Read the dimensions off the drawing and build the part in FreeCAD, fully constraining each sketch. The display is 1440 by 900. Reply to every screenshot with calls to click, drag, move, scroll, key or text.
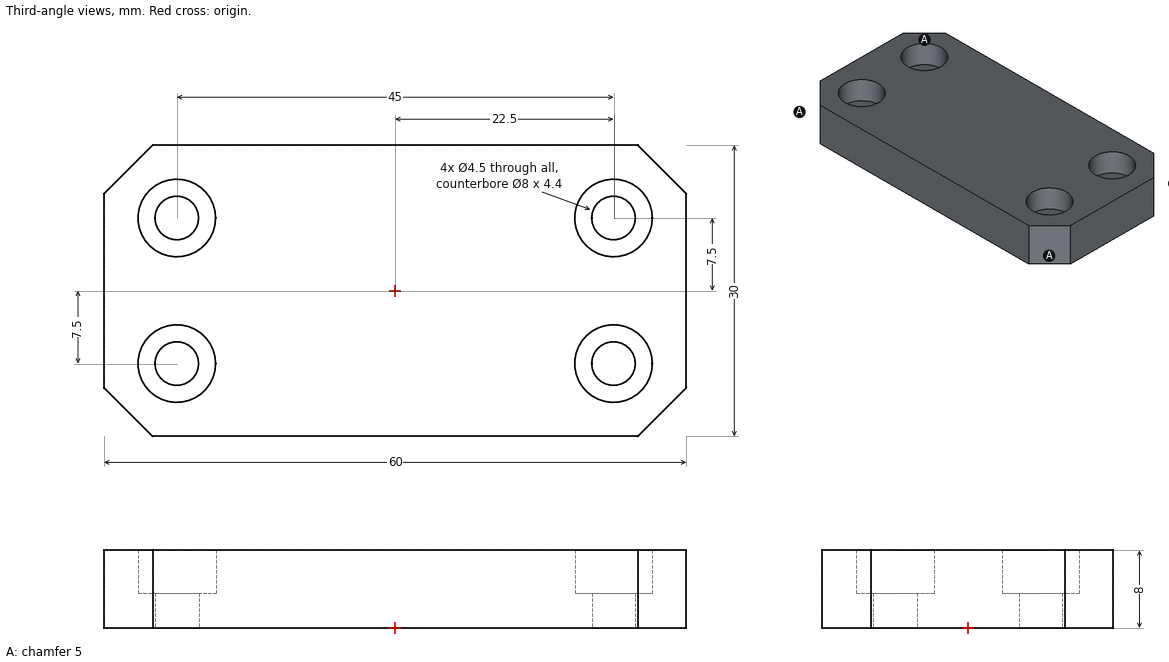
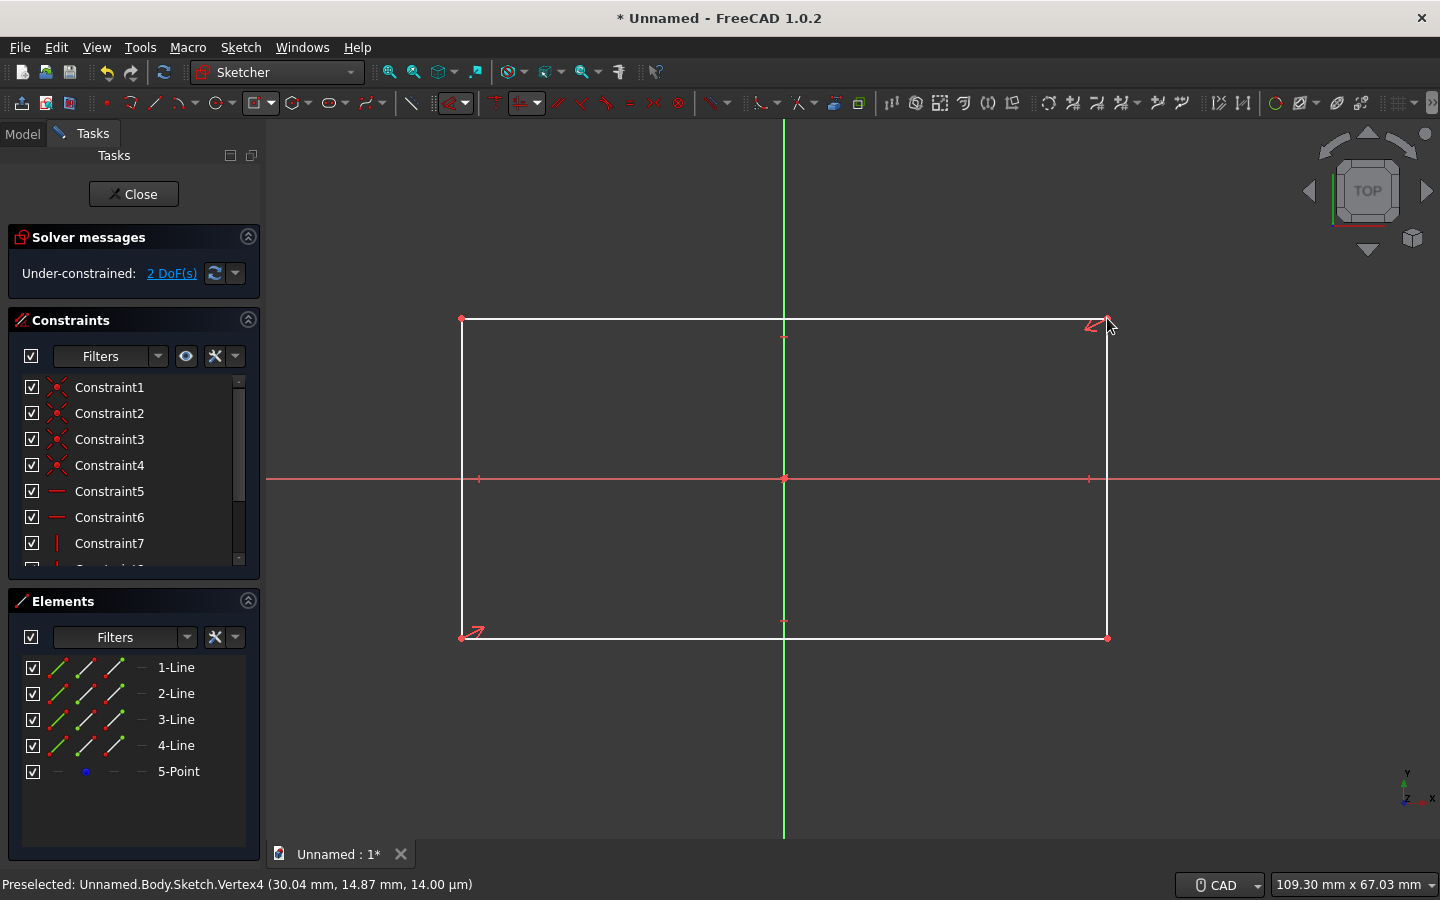
click(450, 104)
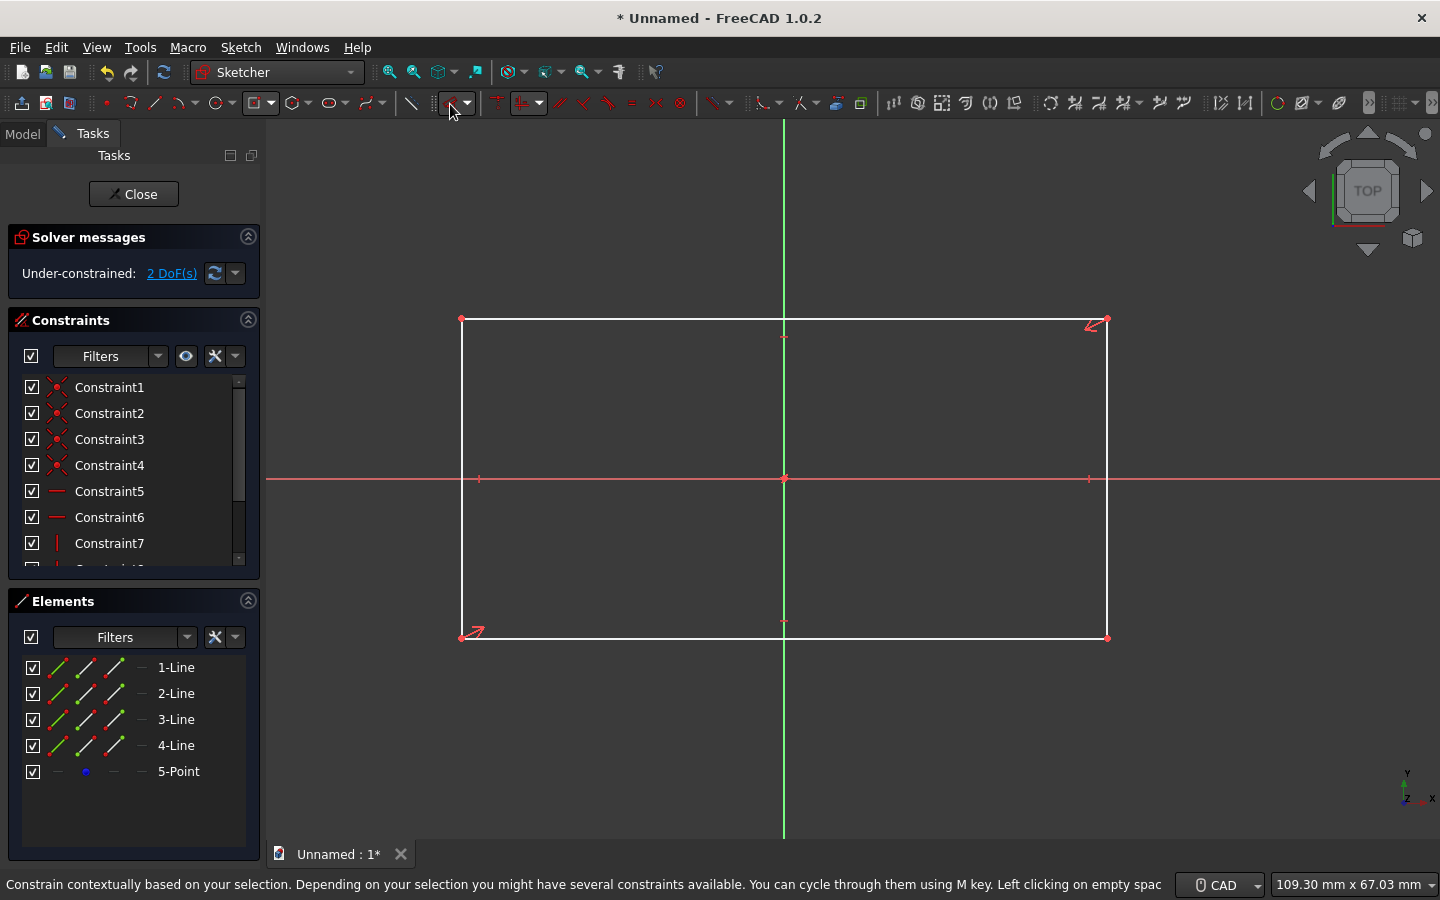
click(655, 639)
click(636, 673)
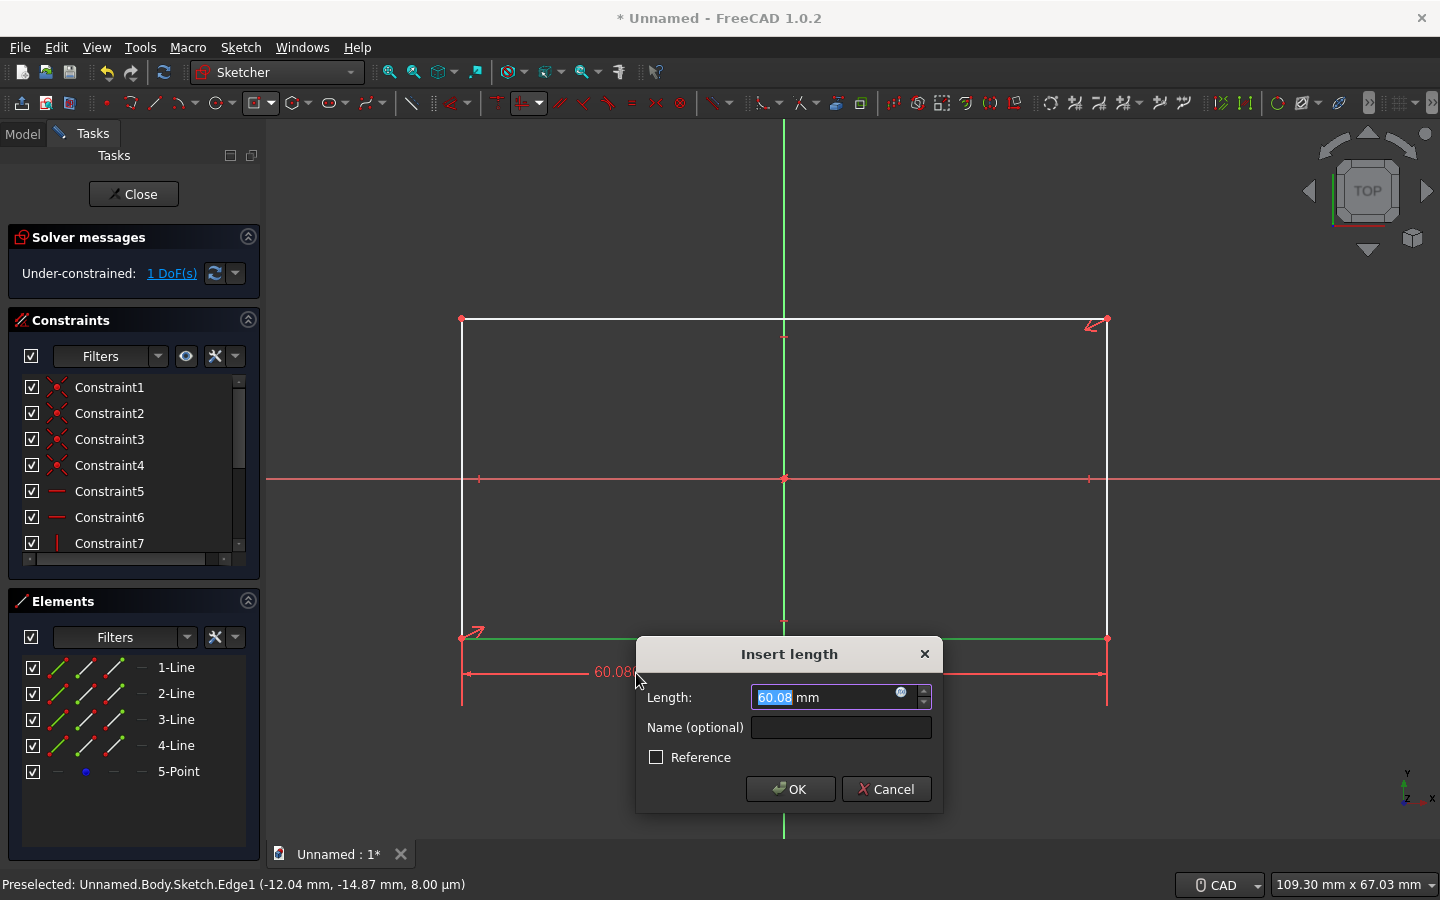
text(60)
key(Return)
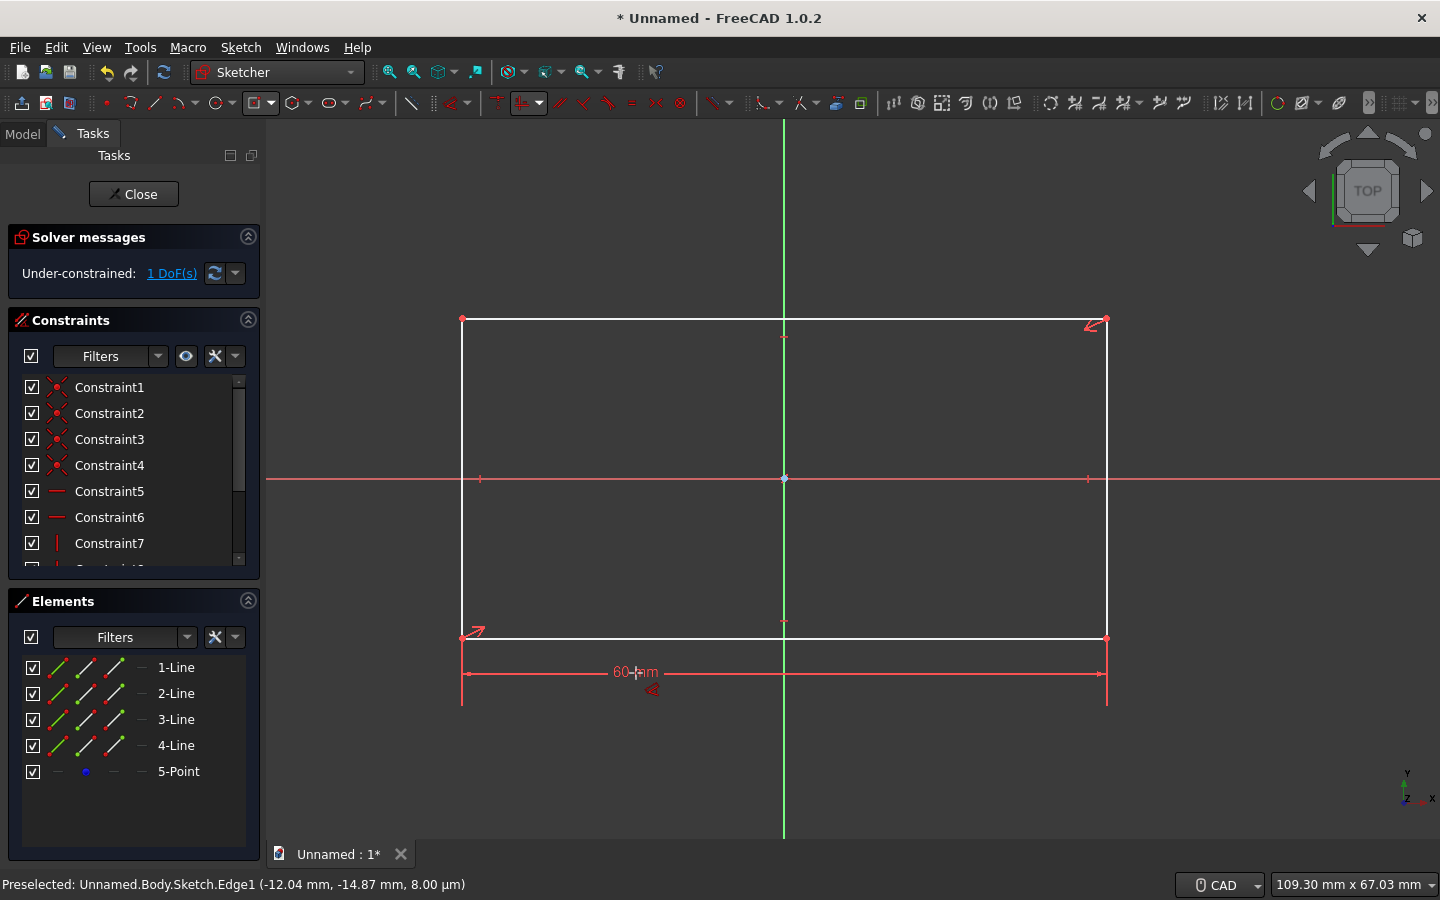
click(1107, 543)
click(1141, 405)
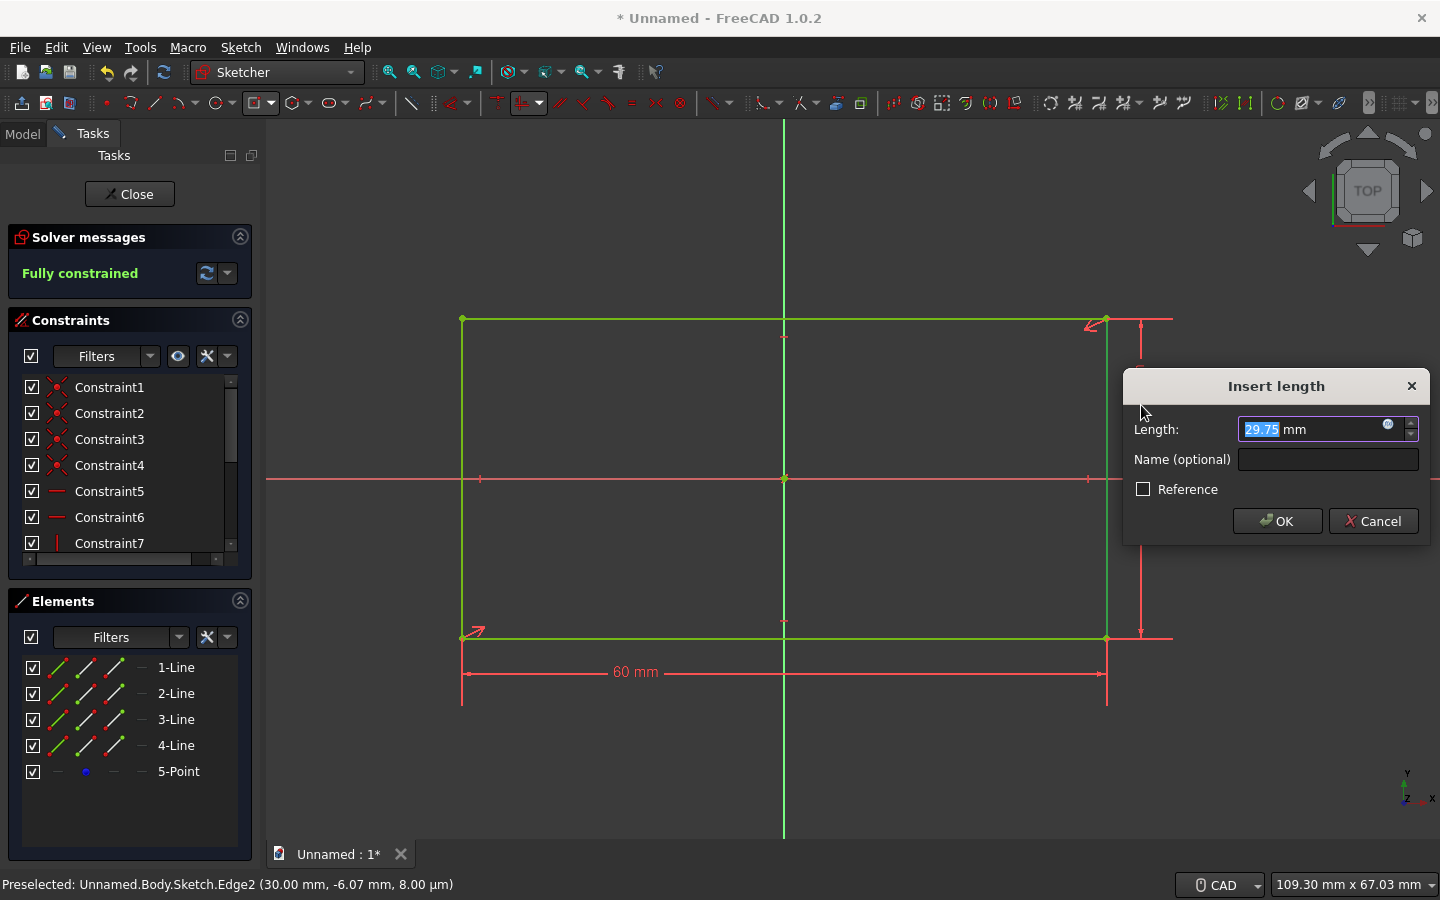
text(30)
key(Return)
key(Escape)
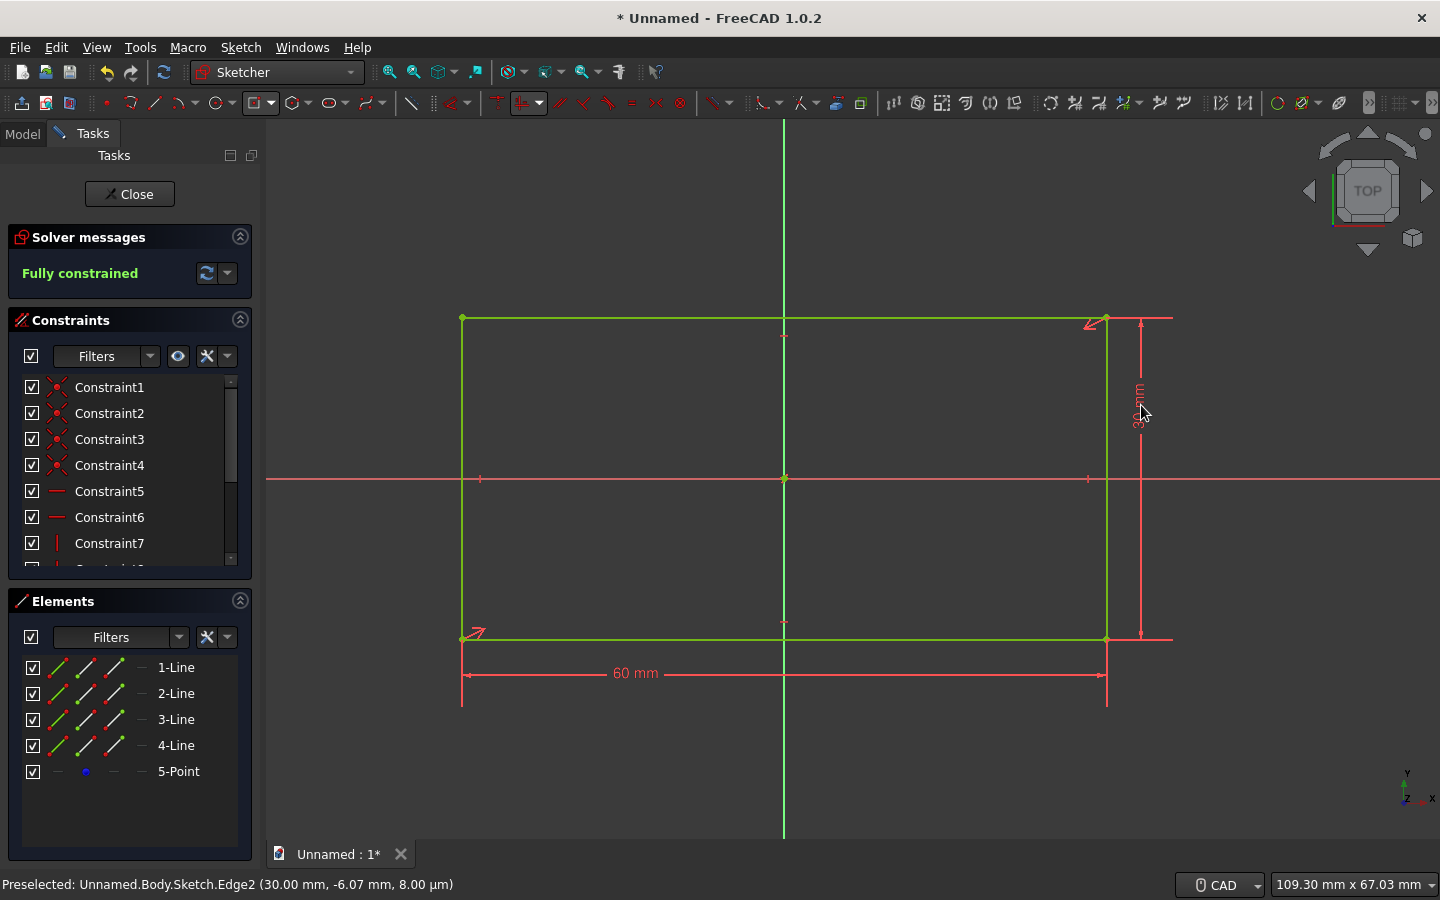
click(130, 194)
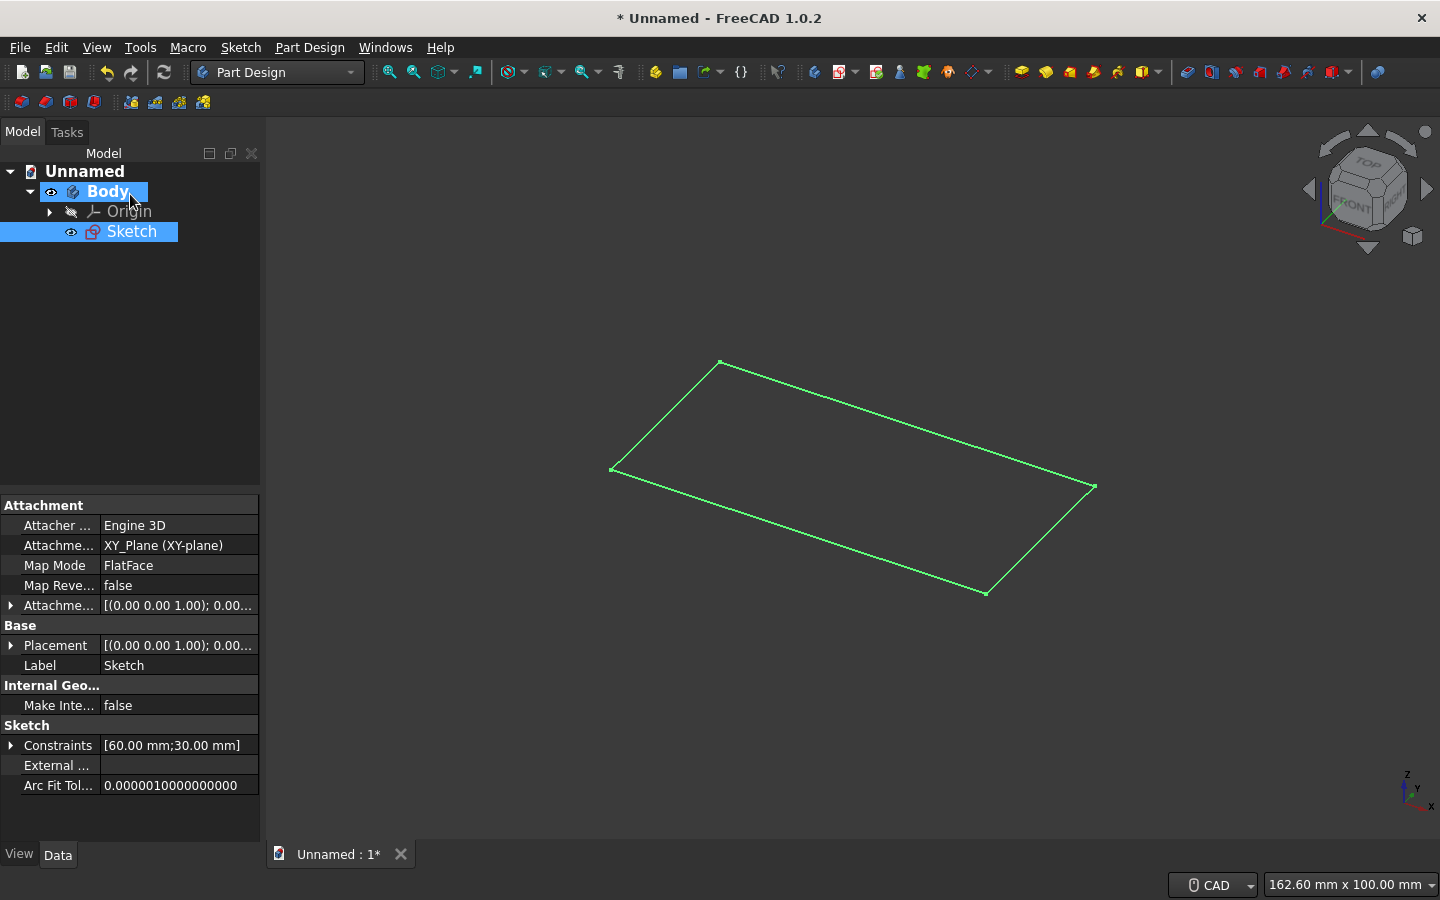
click(1022, 72)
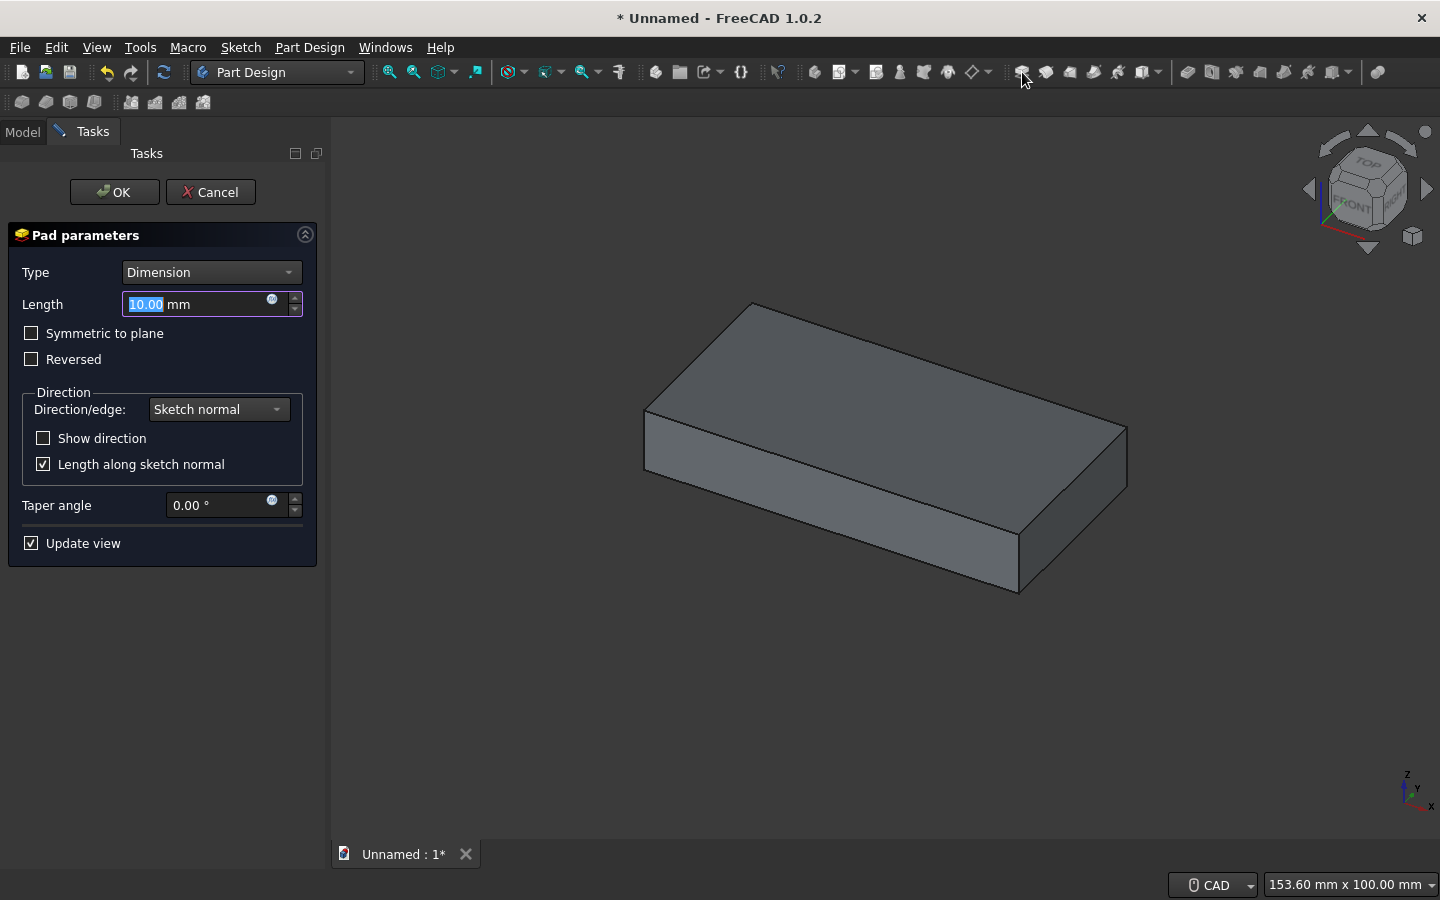
text(8)
key(Tab)